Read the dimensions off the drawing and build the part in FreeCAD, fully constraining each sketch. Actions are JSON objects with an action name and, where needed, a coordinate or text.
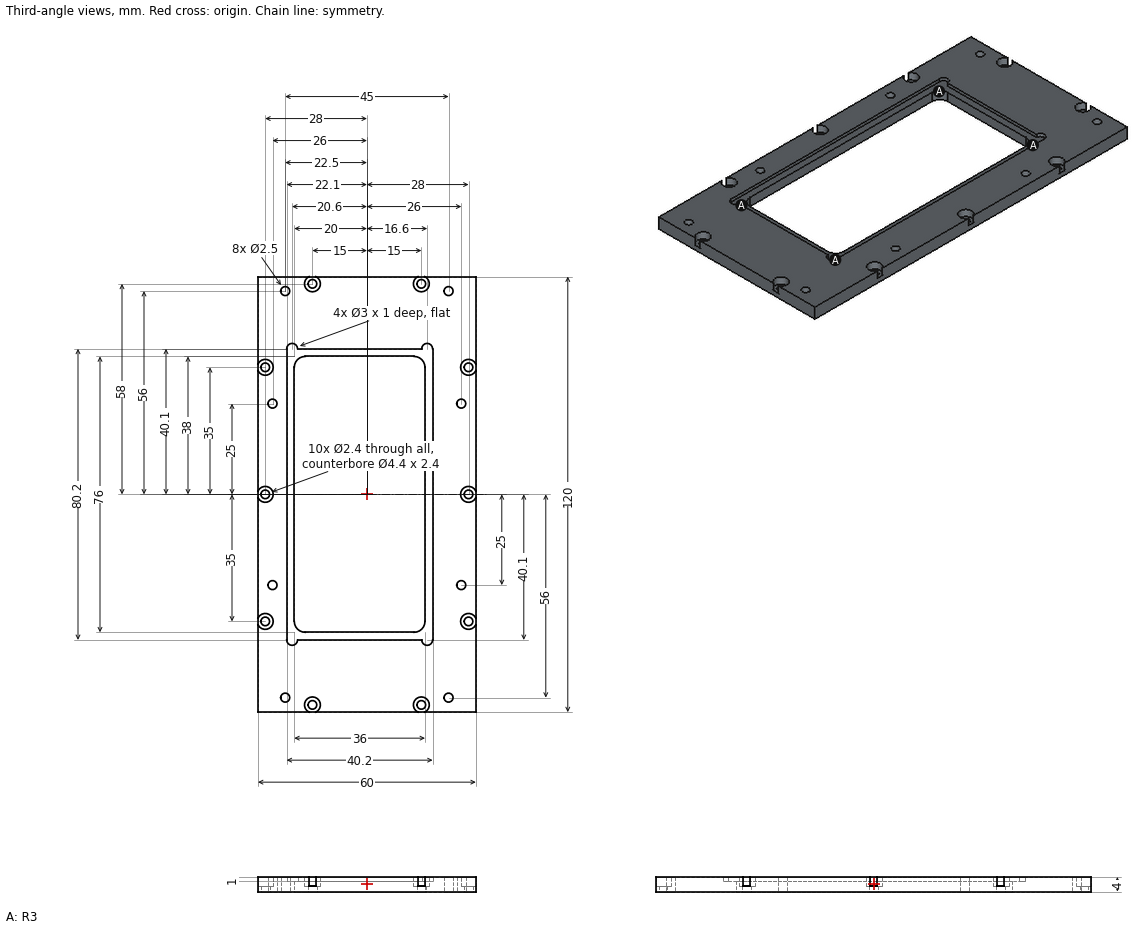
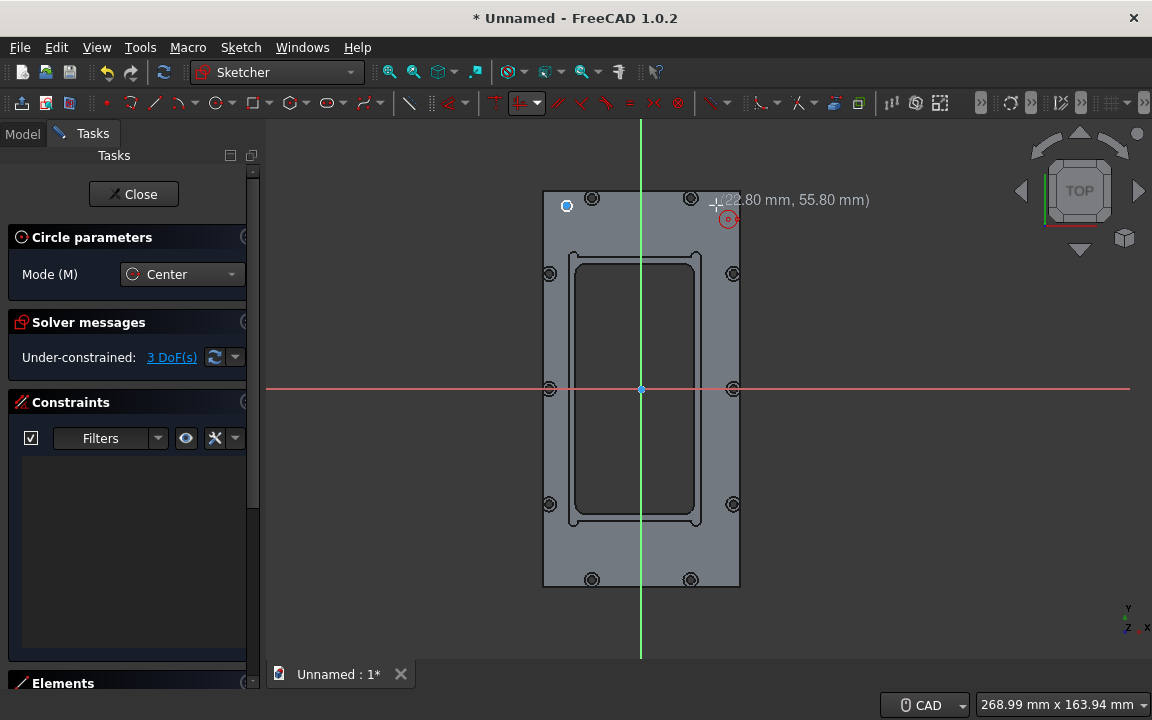
{"action": "left_click", "coordinate": [715, 205]}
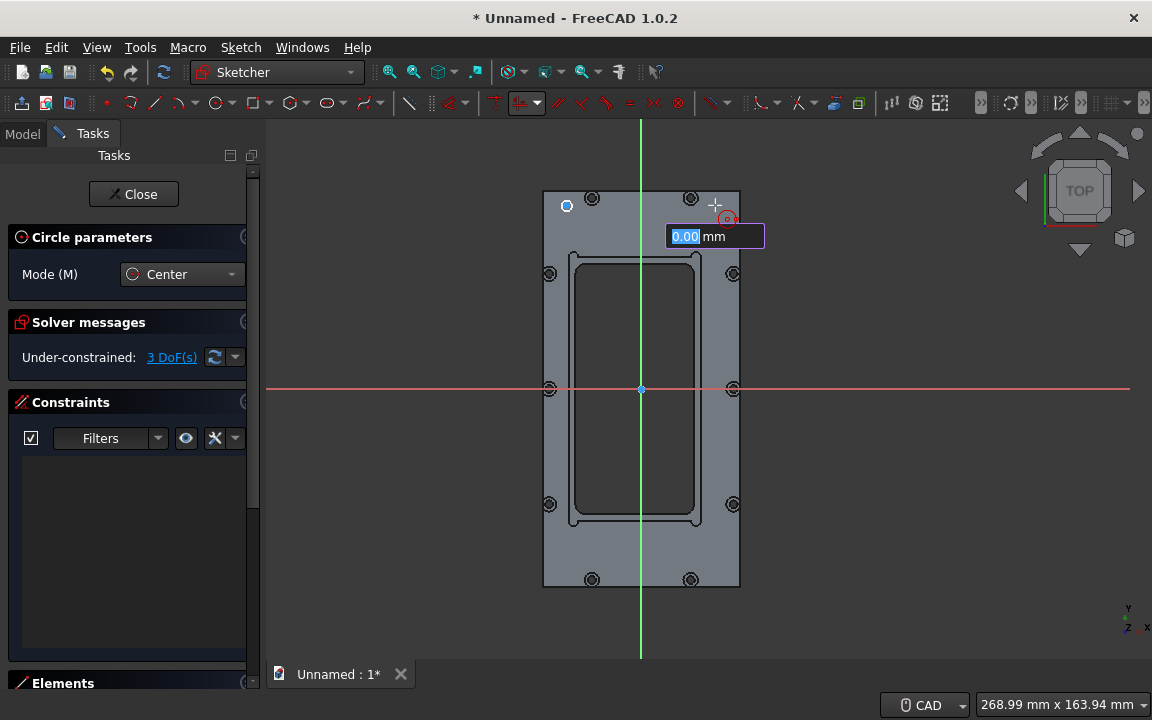
{"action": "scroll", "coordinate": [718, 202], "scroll_direction": "up", "scroll_amount": 7}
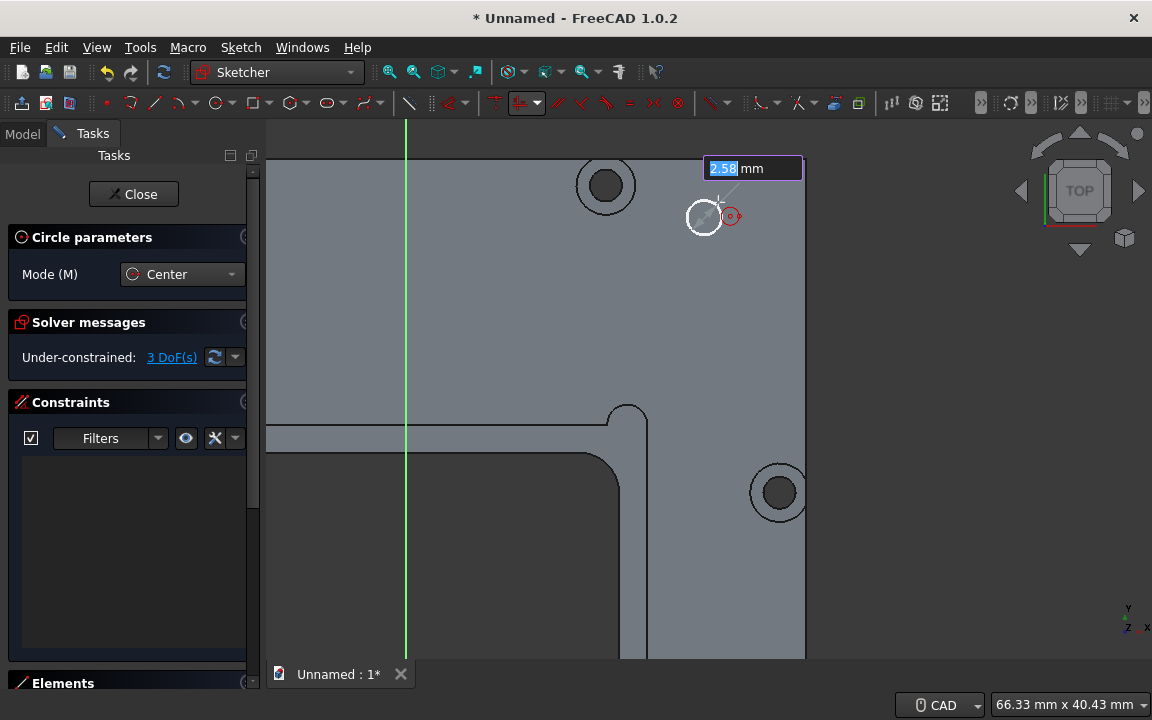
{"action": "left_click", "coordinate": [718, 200]}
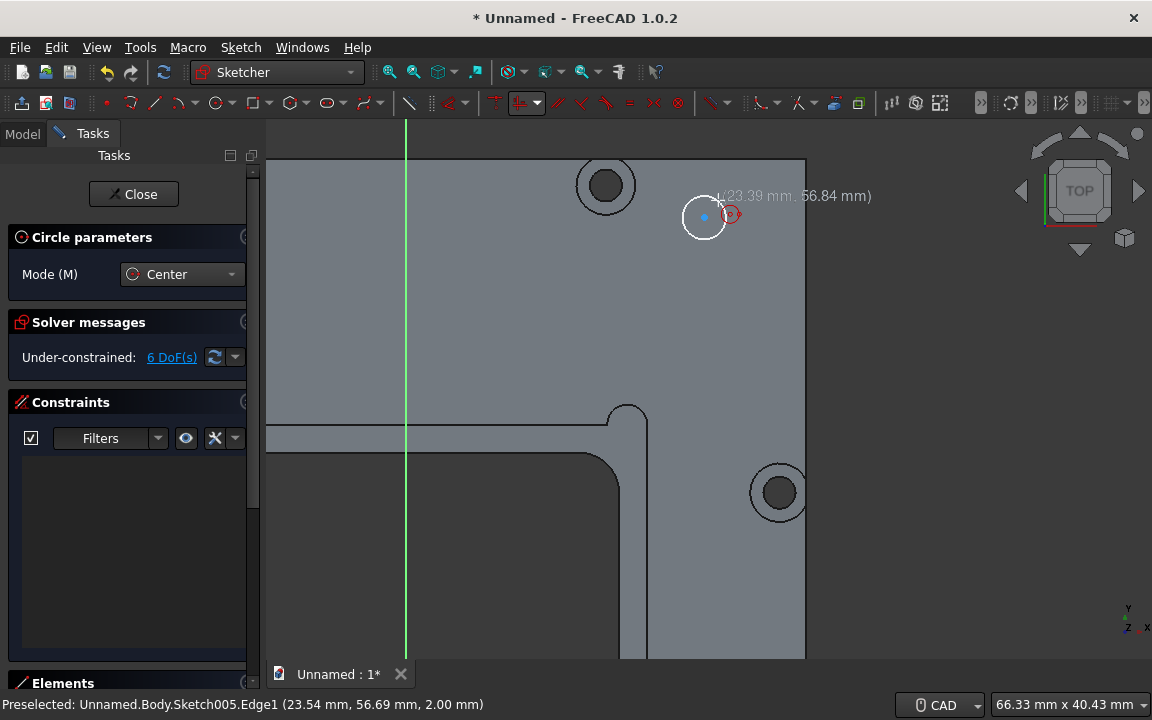
{"action": "scroll", "coordinate": [717, 202], "scroll_direction": "down", "scroll_amount": 7}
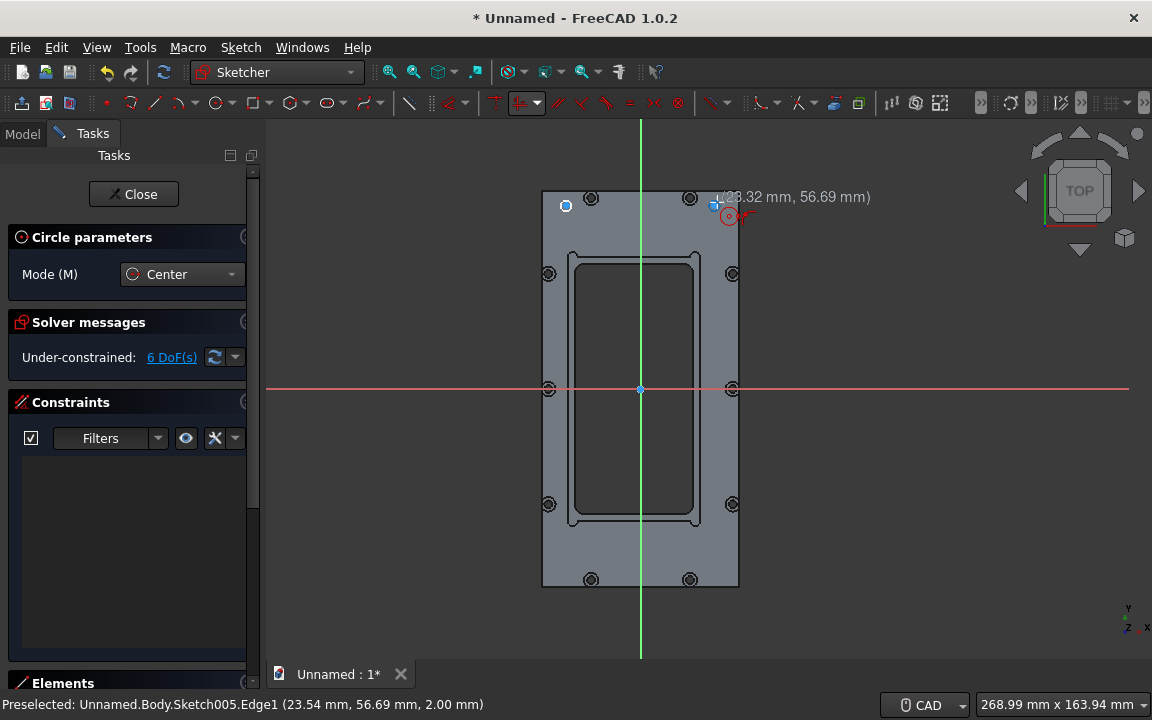
{"action": "scroll", "coordinate": [555, 307], "scroll_direction": "up", "scroll_amount": 9}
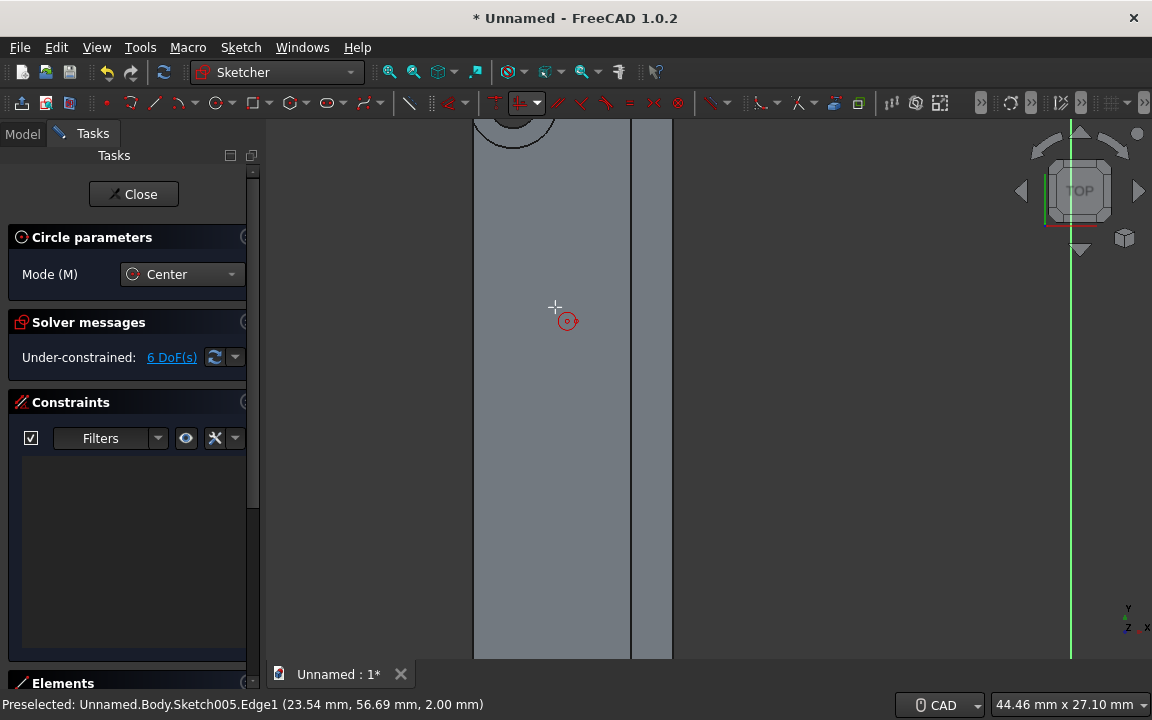
{"action": "scroll", "coordinate": [555, 307], "scroll_direction": "down", "scroll_amount": 9}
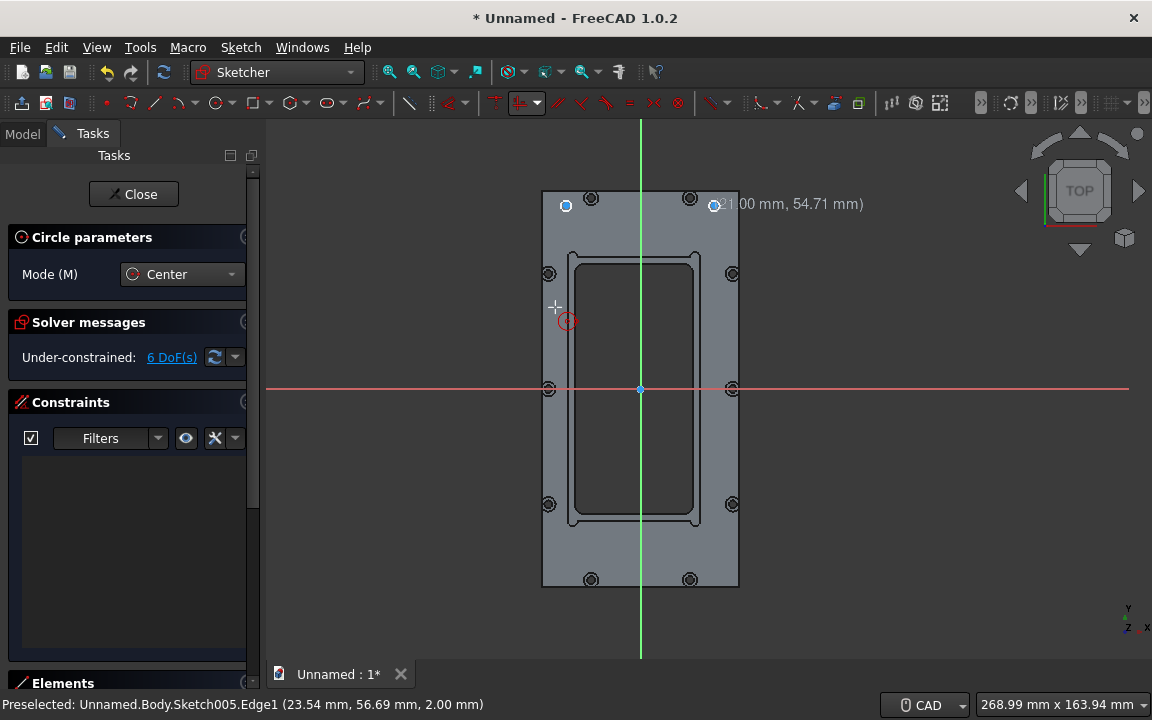
{"action": "left_click", "coordinate": [555, 307]}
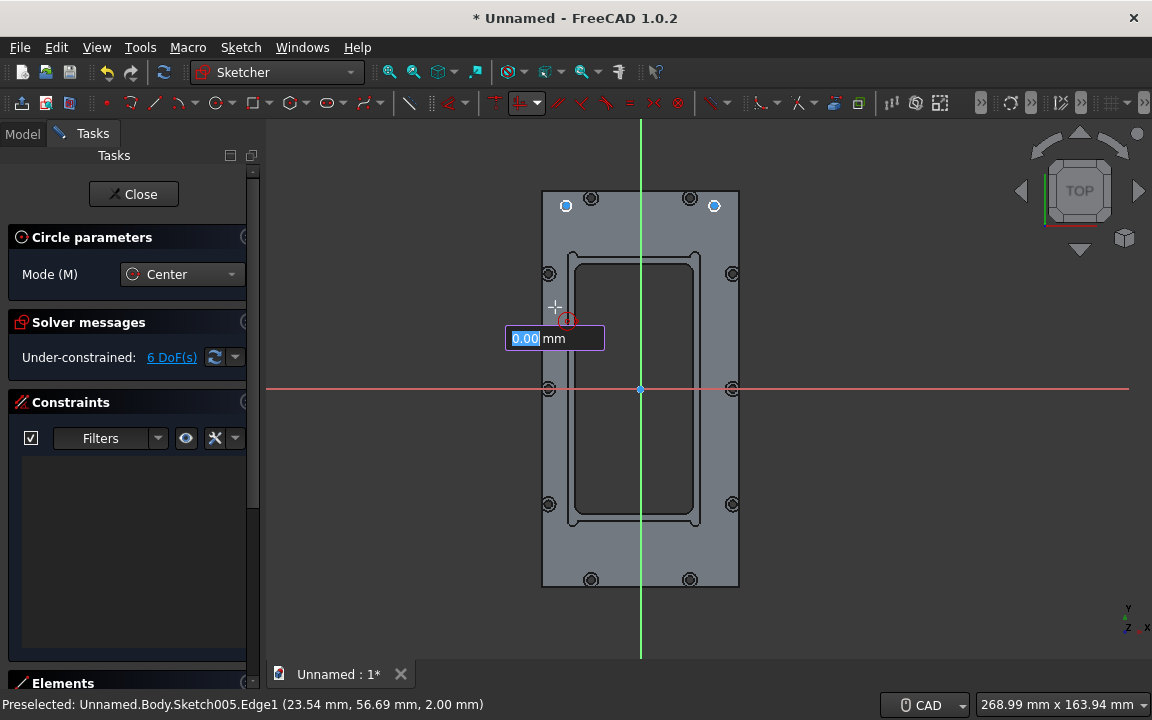
{"action": "scroll", "coordinate": [558, 304], "scroll_direction": "up", "scroll_amount": 7}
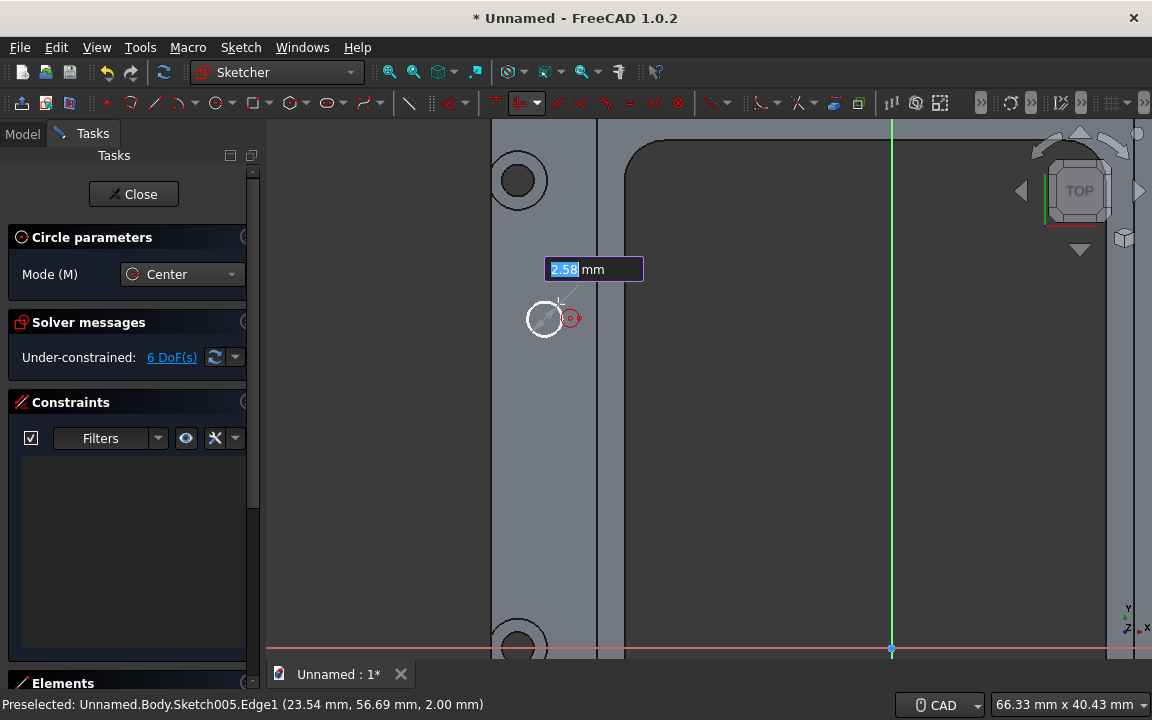
{"action": "left_click", "coordinate": [556, 302]}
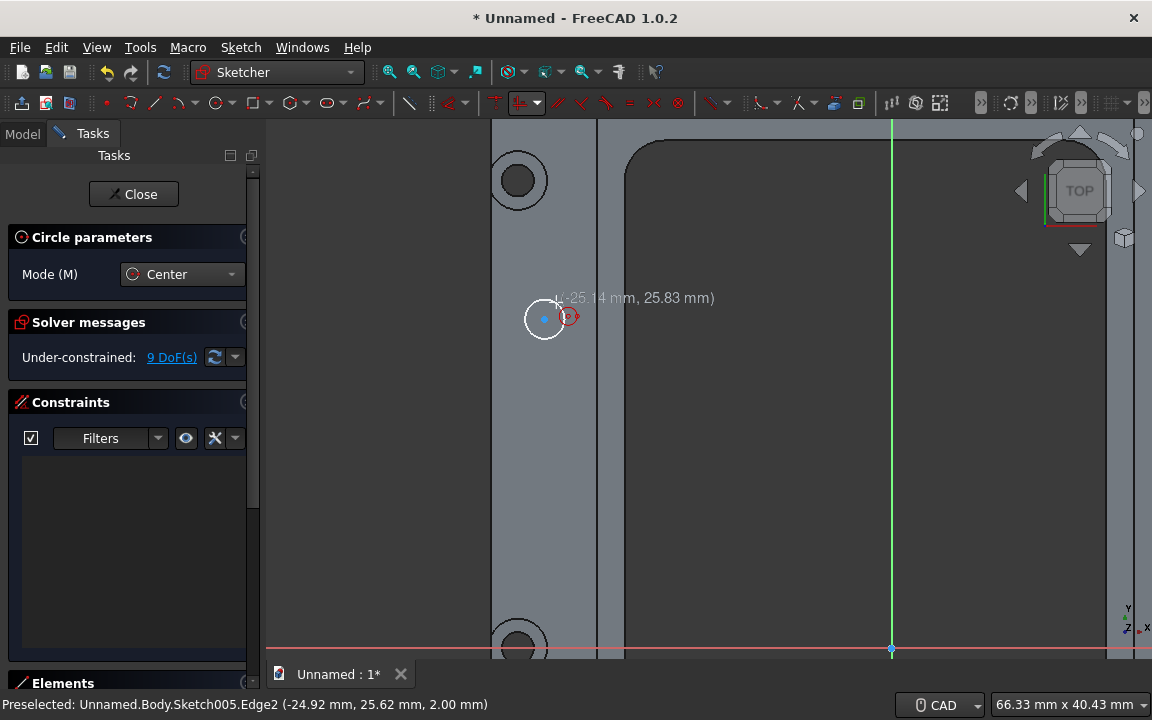
{"action": "scroll", "coordinate": [558, 304], "scroll_direction": "down", "scroll_amount": 7}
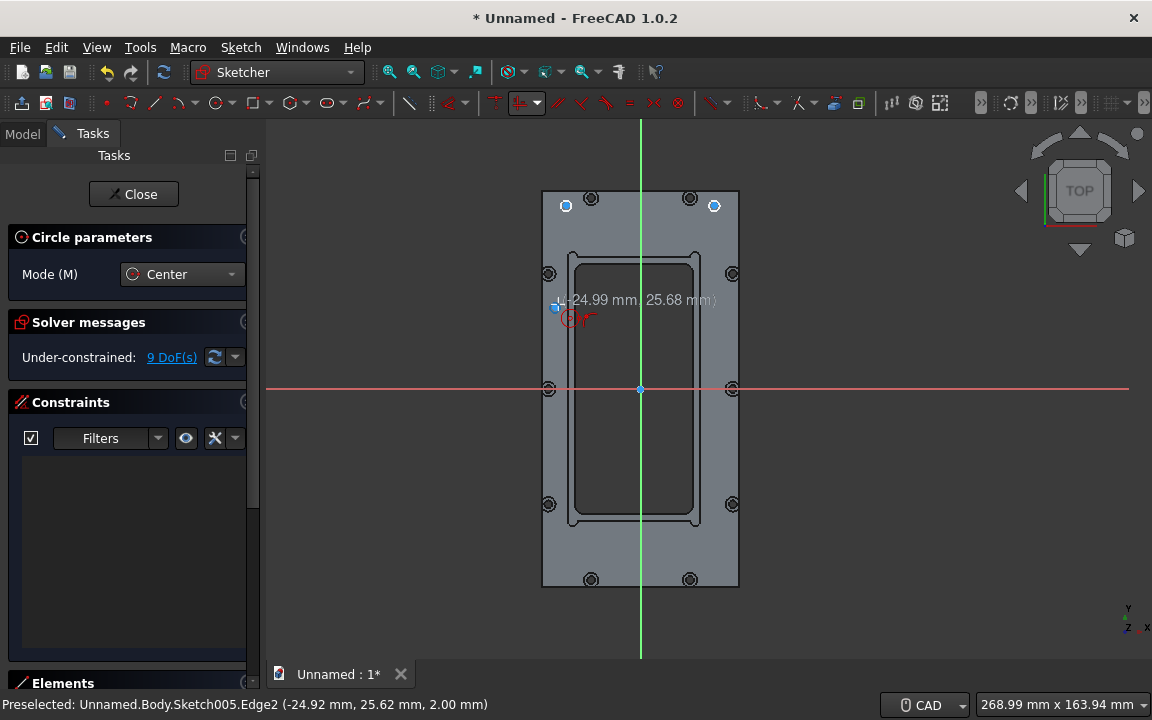
{"action": "scroll", "coordinate": [726, 307], "scroll_direction": "up", "scroll_amount": 9}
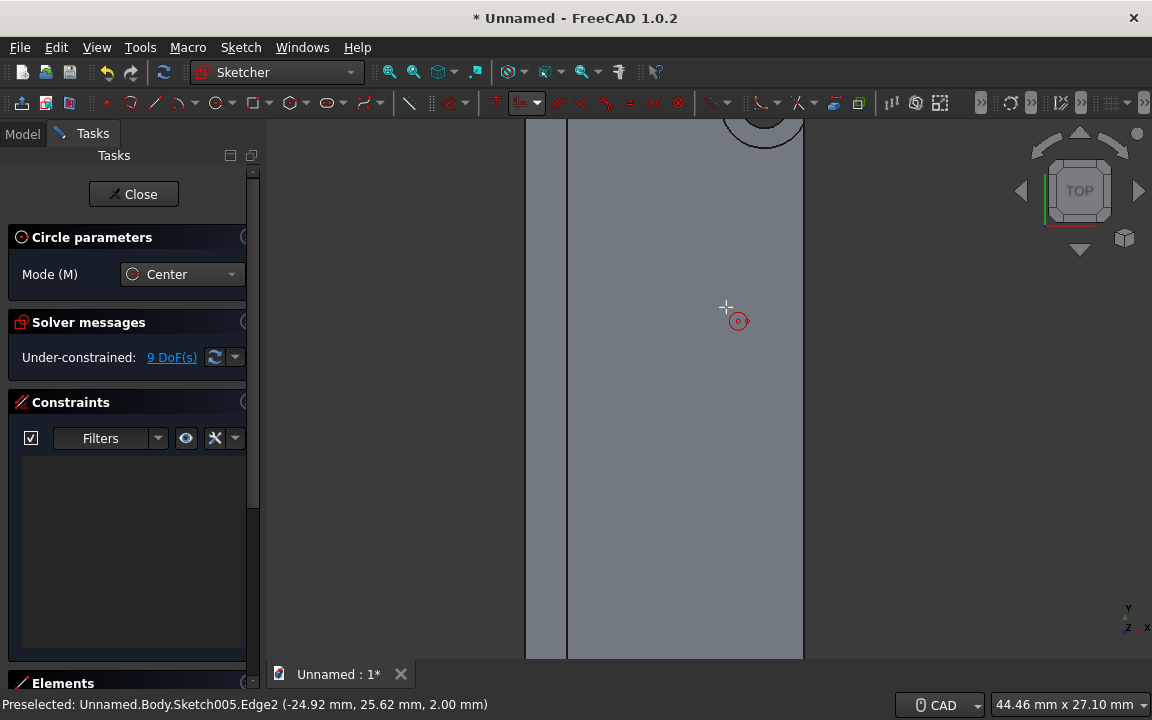
{"action": "scroll", "coordinate": [726, 307], "scroll_direction": "down", "scroll_amount": 9}